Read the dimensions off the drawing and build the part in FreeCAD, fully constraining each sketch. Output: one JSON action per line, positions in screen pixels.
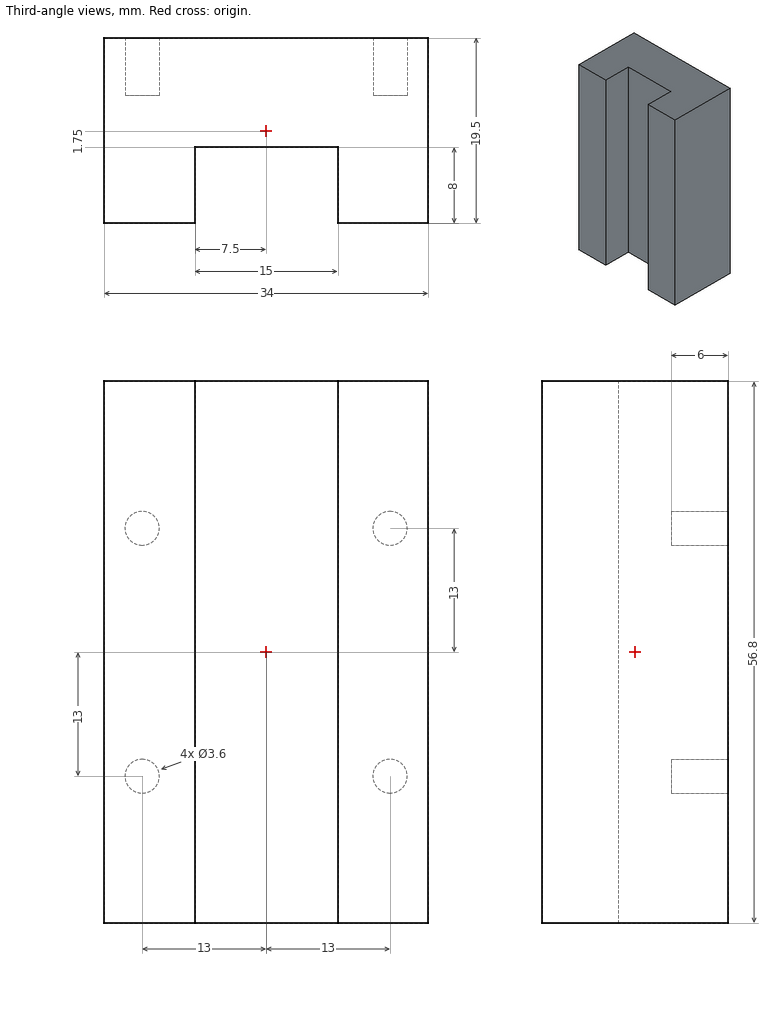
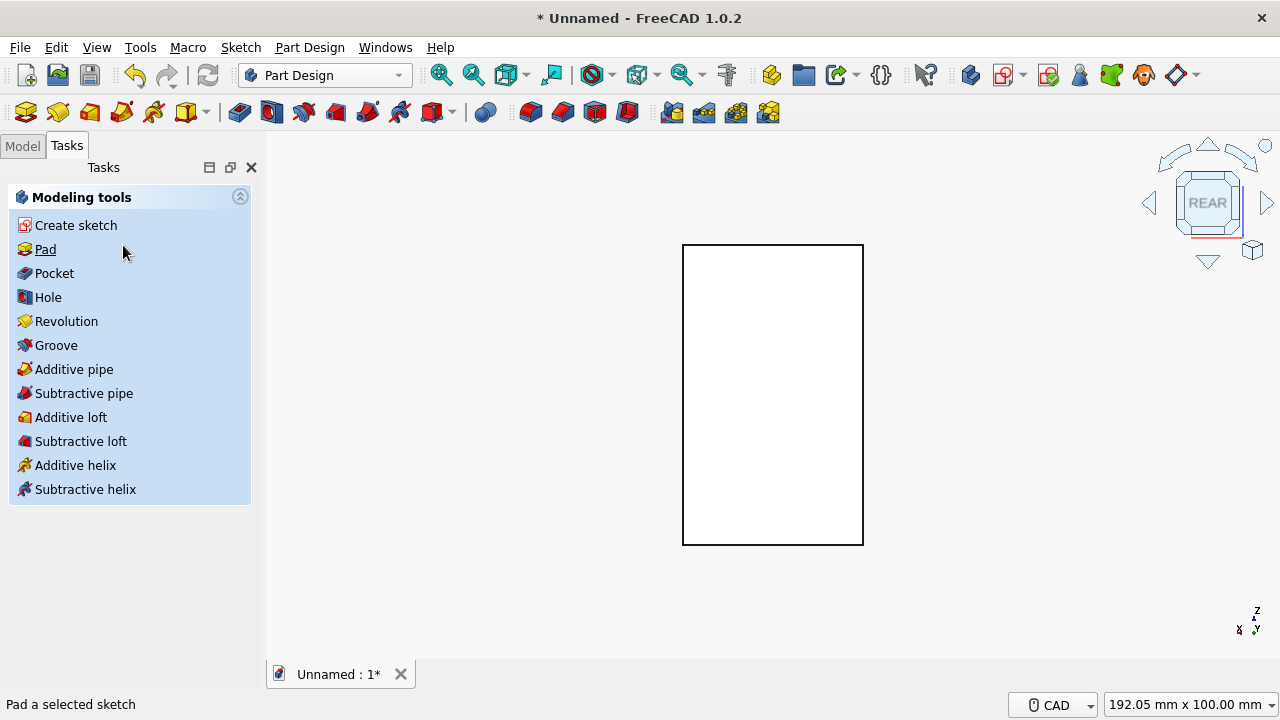
{"action": "left_click", "coordinate": [240, 112]}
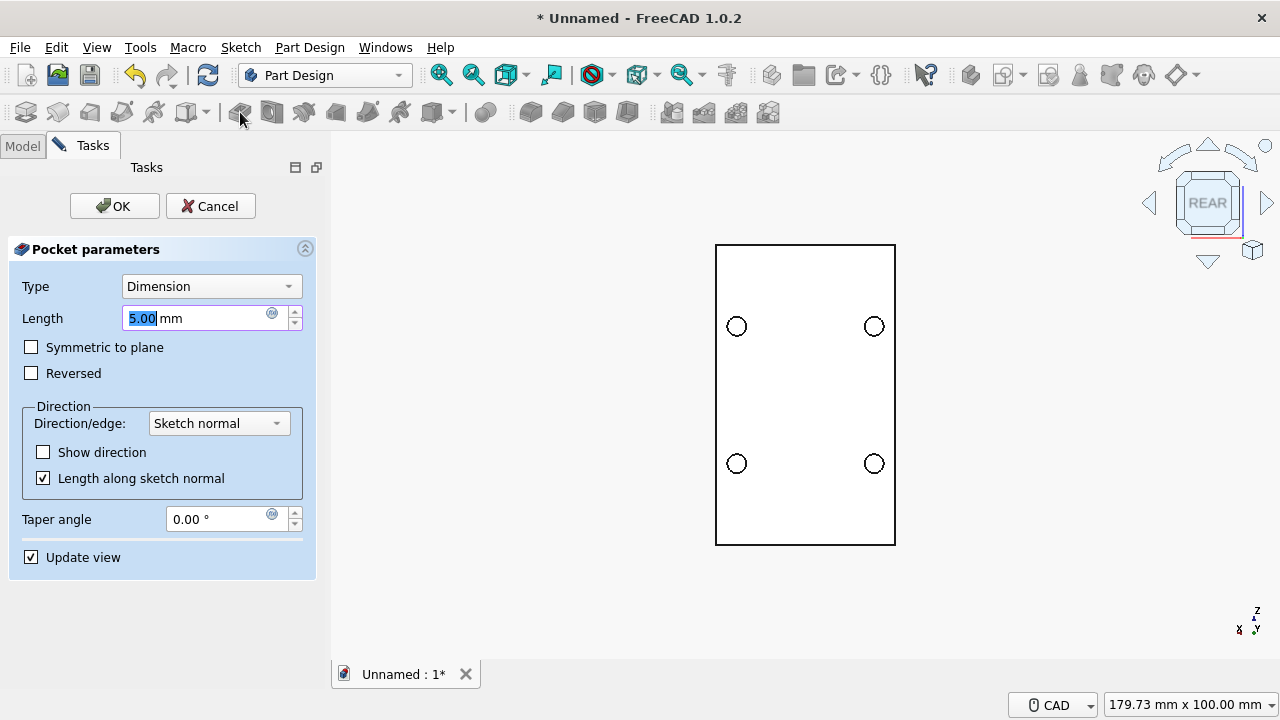
{"action": "type", "text": "6"}
{"action": "key", "text": "Tab"}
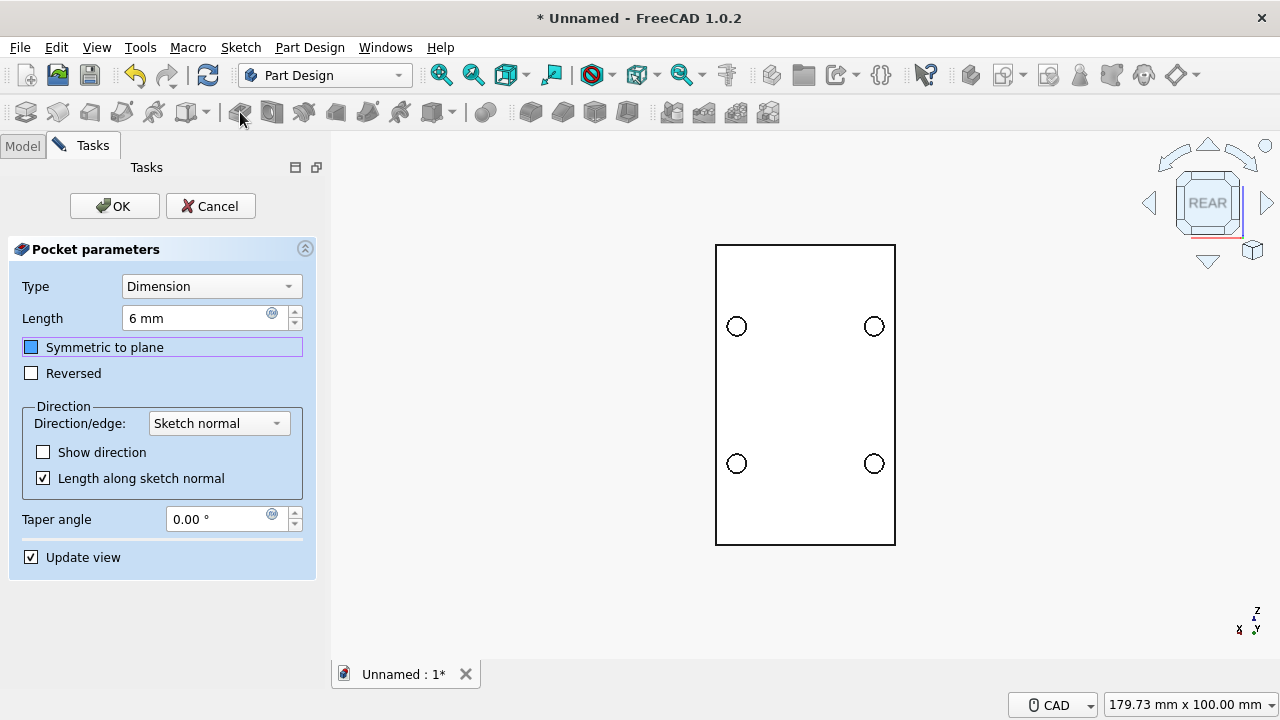
{"action": "left_click", "coordinate": [115, 206]}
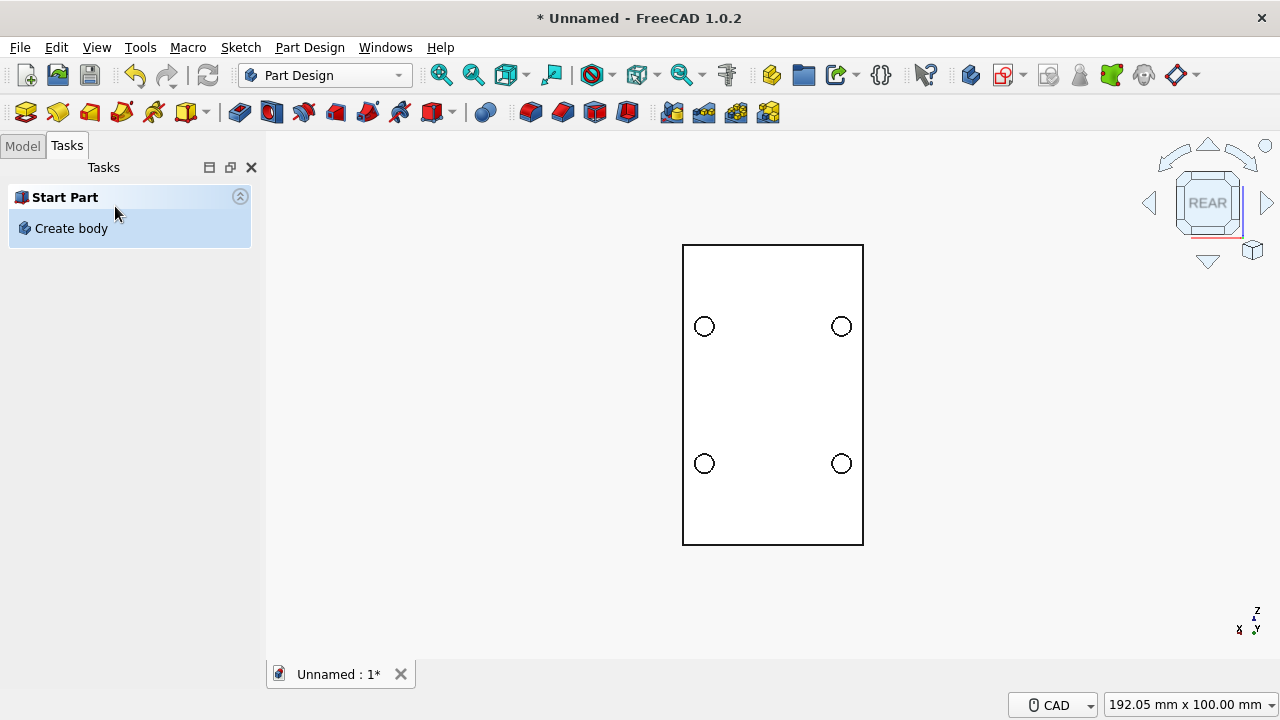
{"action": "key", "text": "0"}